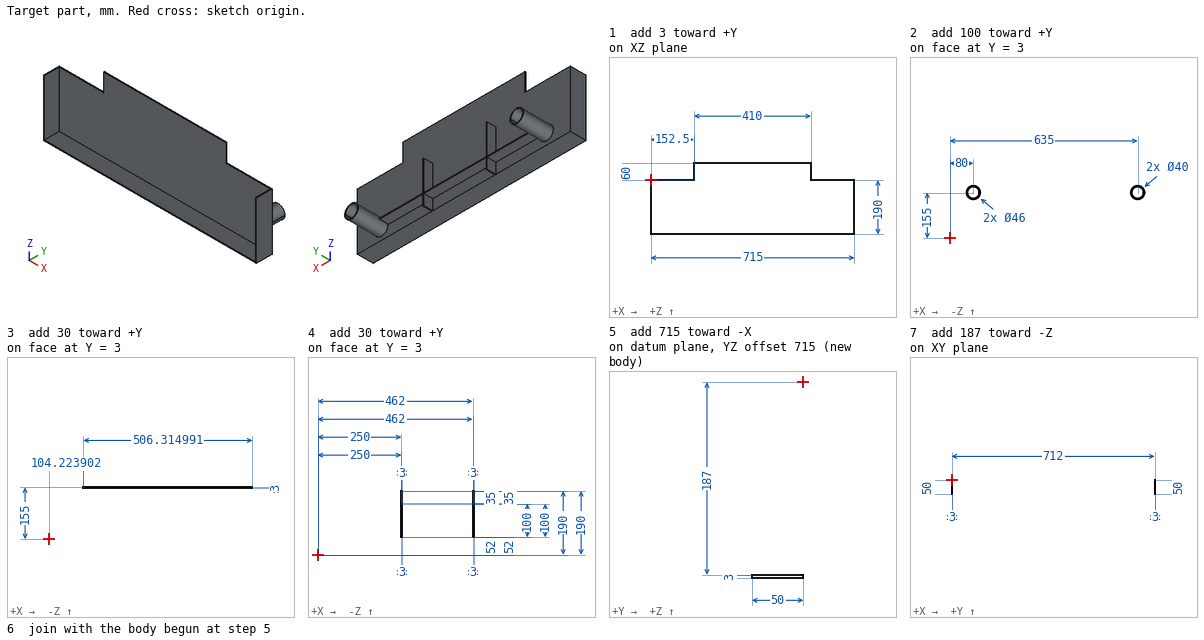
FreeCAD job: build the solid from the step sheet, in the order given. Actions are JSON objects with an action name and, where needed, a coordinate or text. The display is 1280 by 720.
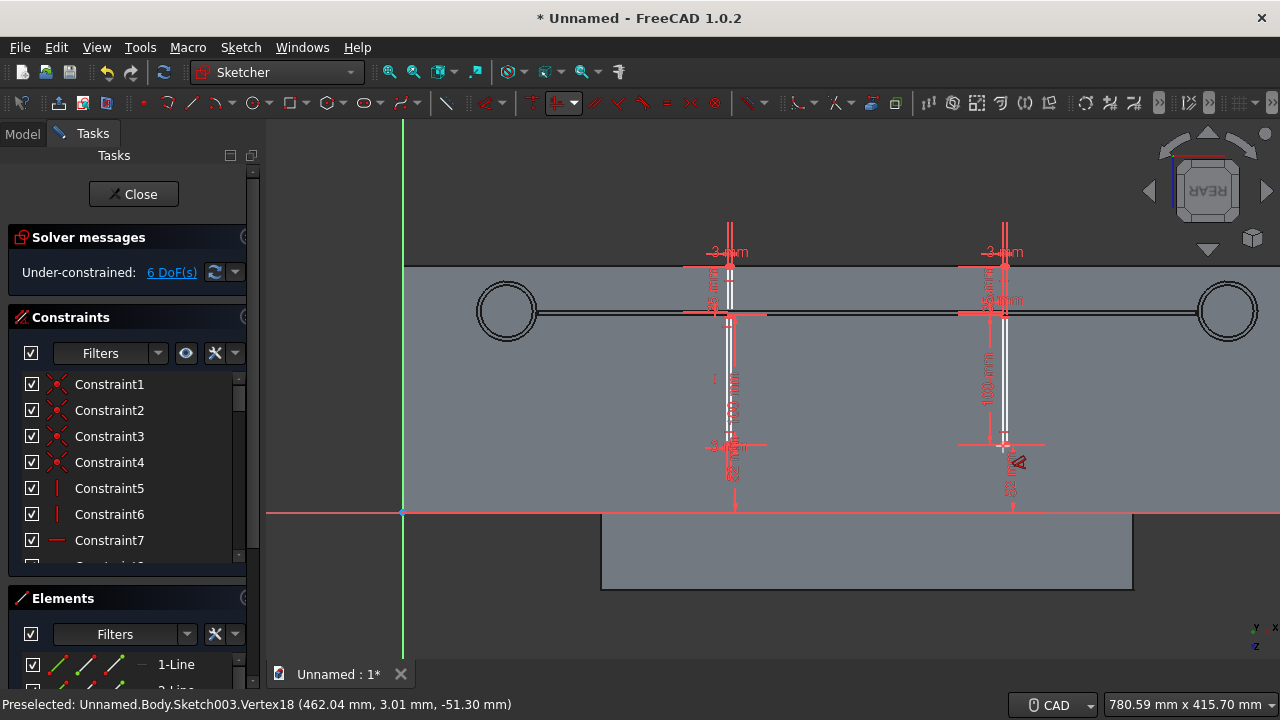
{"action": "scroll", "coordinate": [728, 267], "scroll_direction": "up", "scroll_amount": 6}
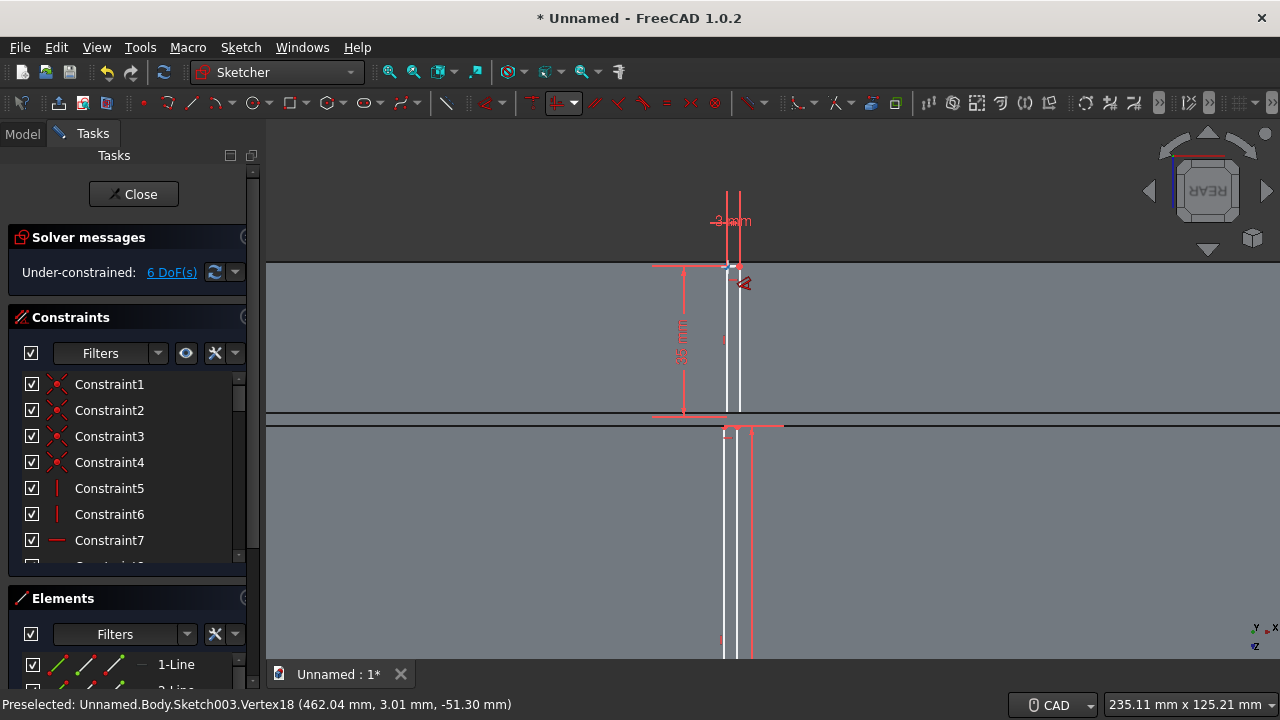
{"action": "left_click", "coordinate": [727, 266]}
{"action": "left_click", "coordinate": [510, 232]}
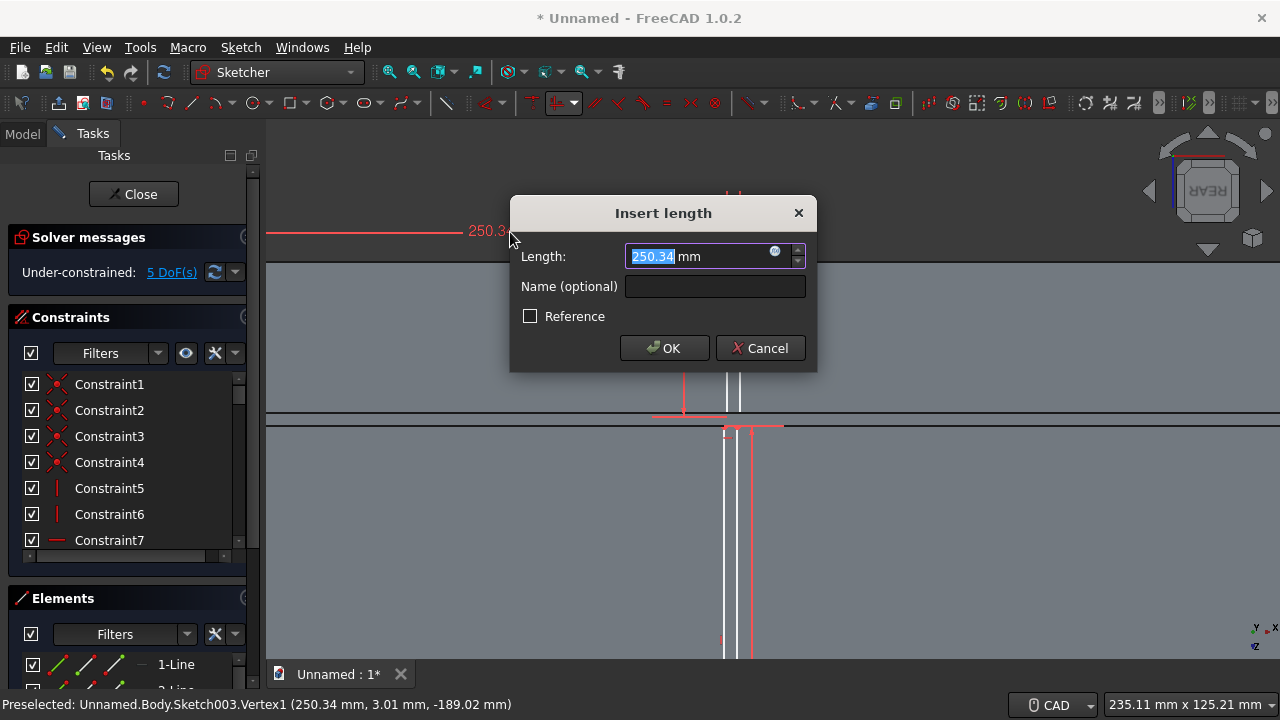
{"action": "type", "text": "250"}
{"action": "key", "text": "Return"}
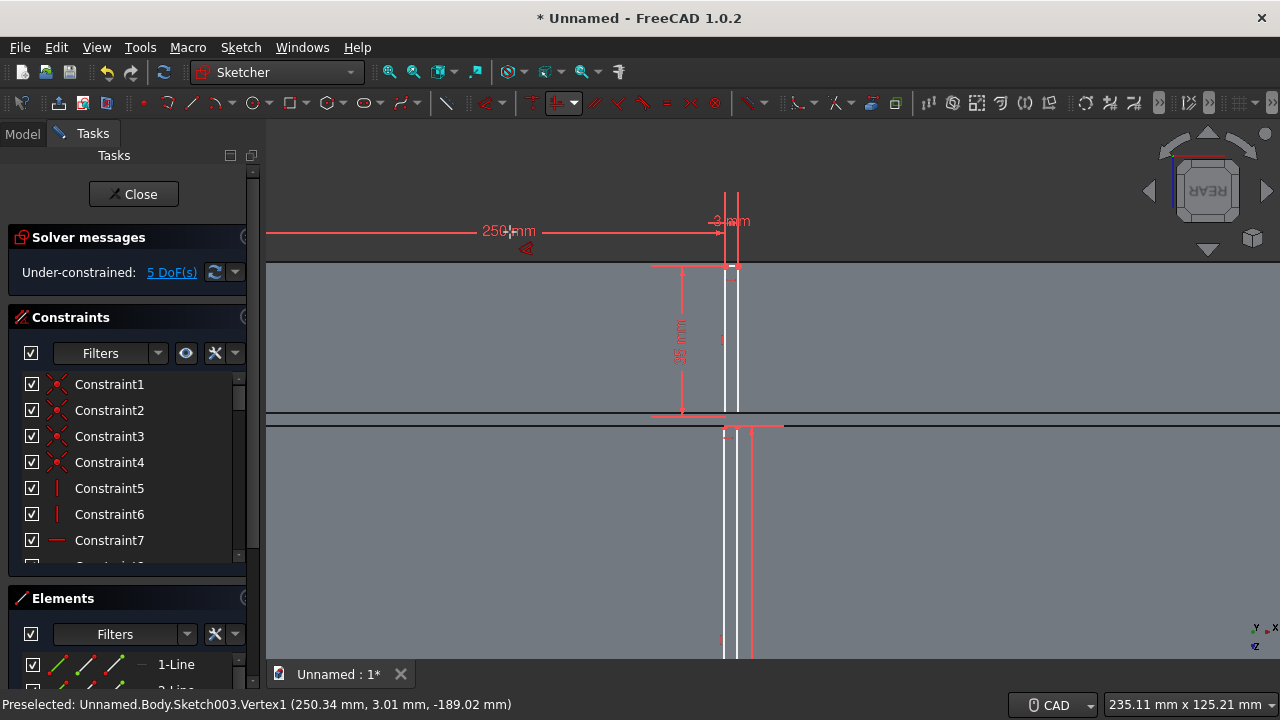
{"action": "left_click", "coordinate": [725, 266]}
{"action": "left_click", "coordinate": [759, 449]}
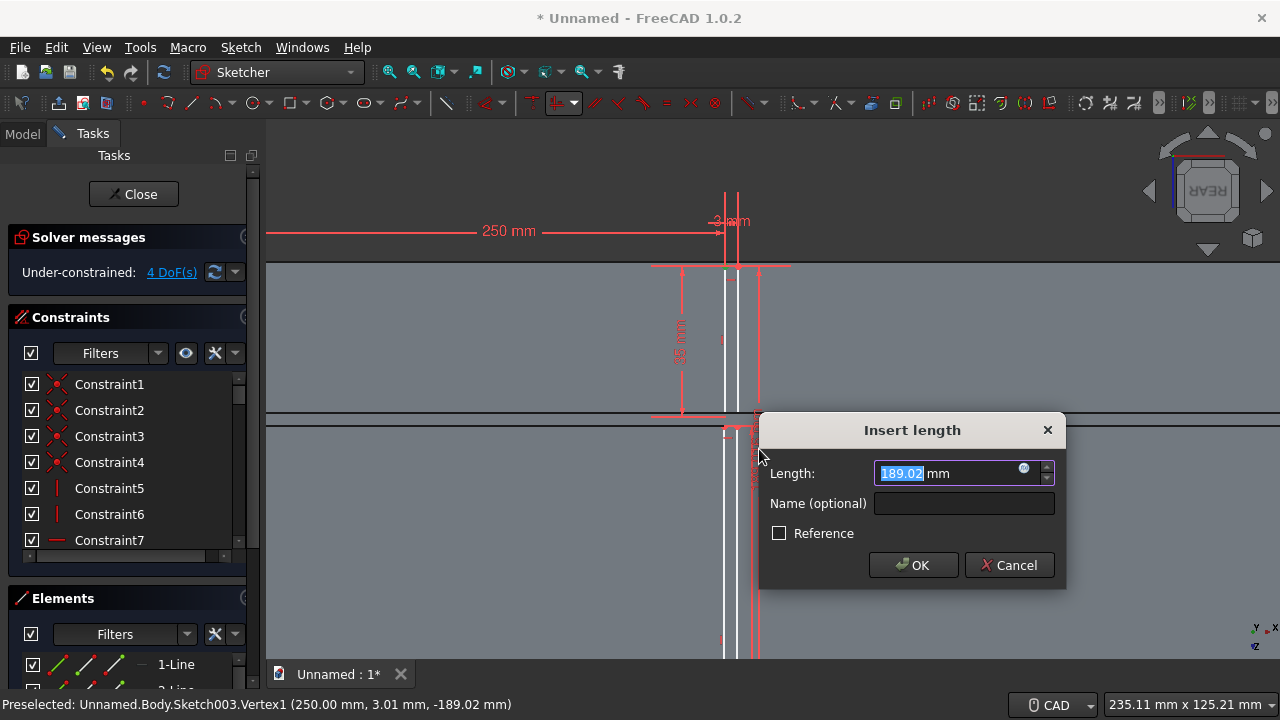
{"action": "type", "text": "190"}
{"action": "key", "text": "Return"}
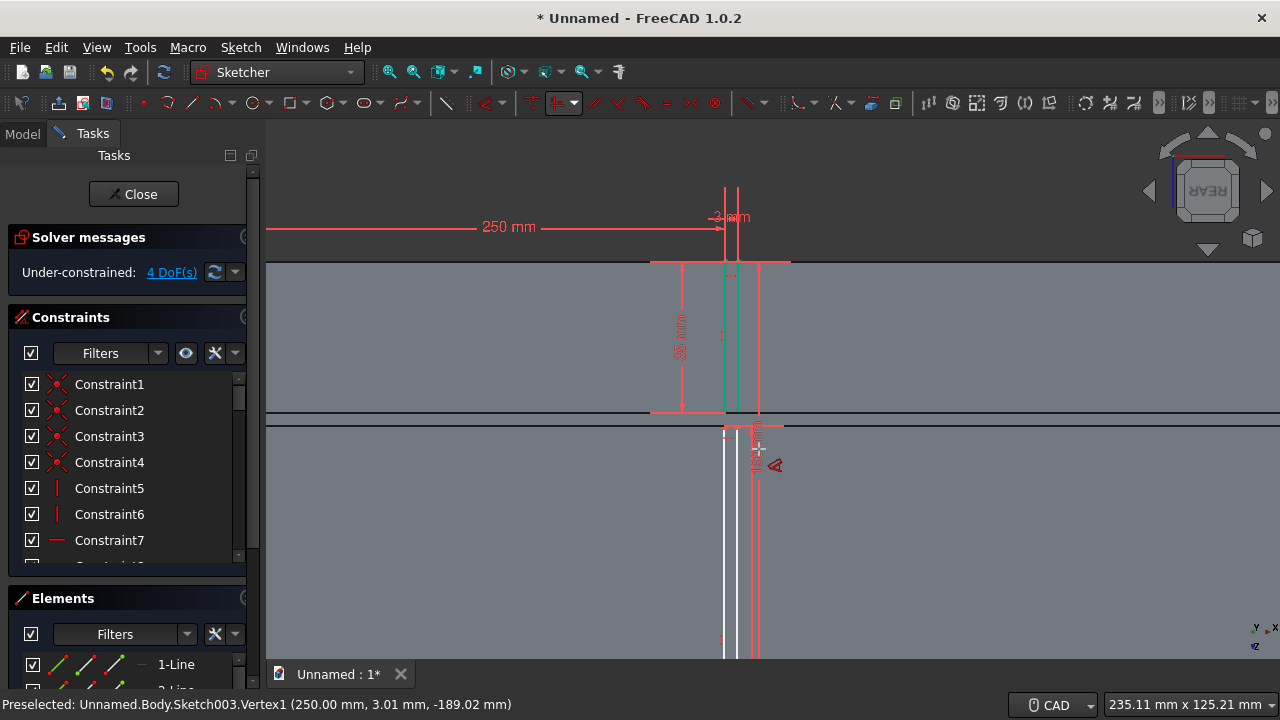
{"action": "left_click", "coordinate": [724, 426]}
{"action": "left_click", "coordinate": [509, 392]}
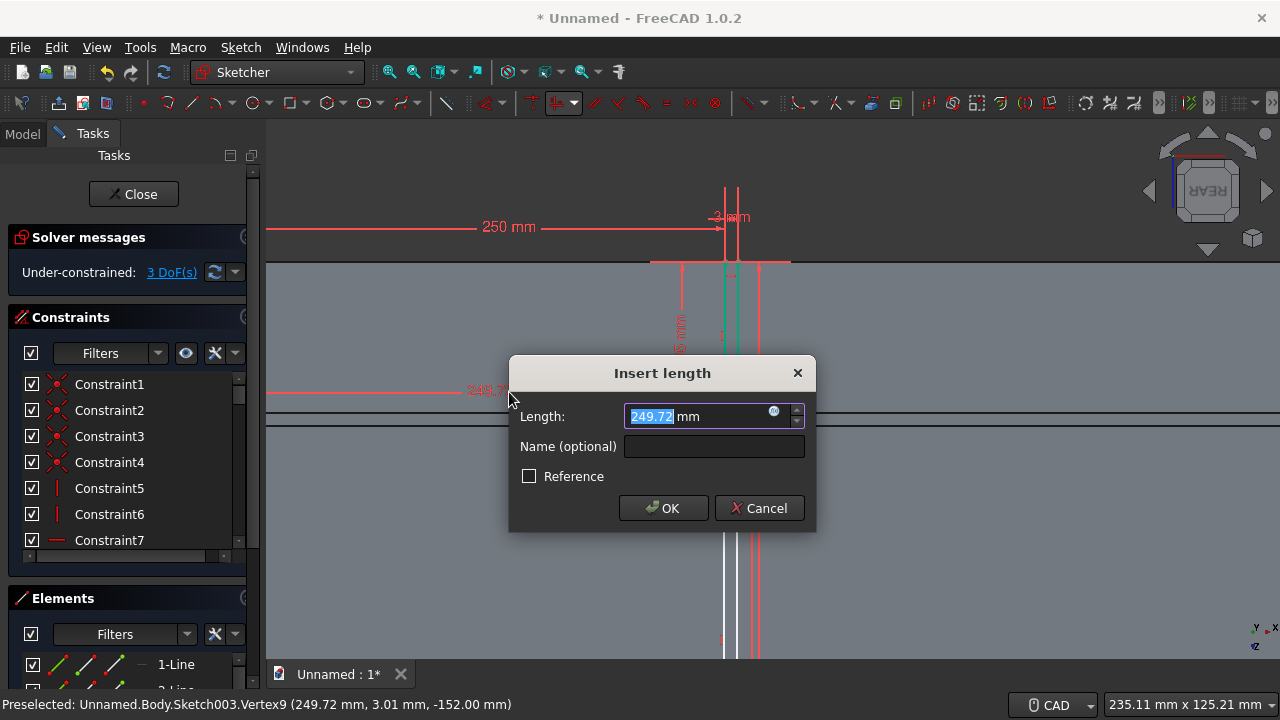
{"action": "type", "text": "250"}
{"action": "key", "text": "Return"}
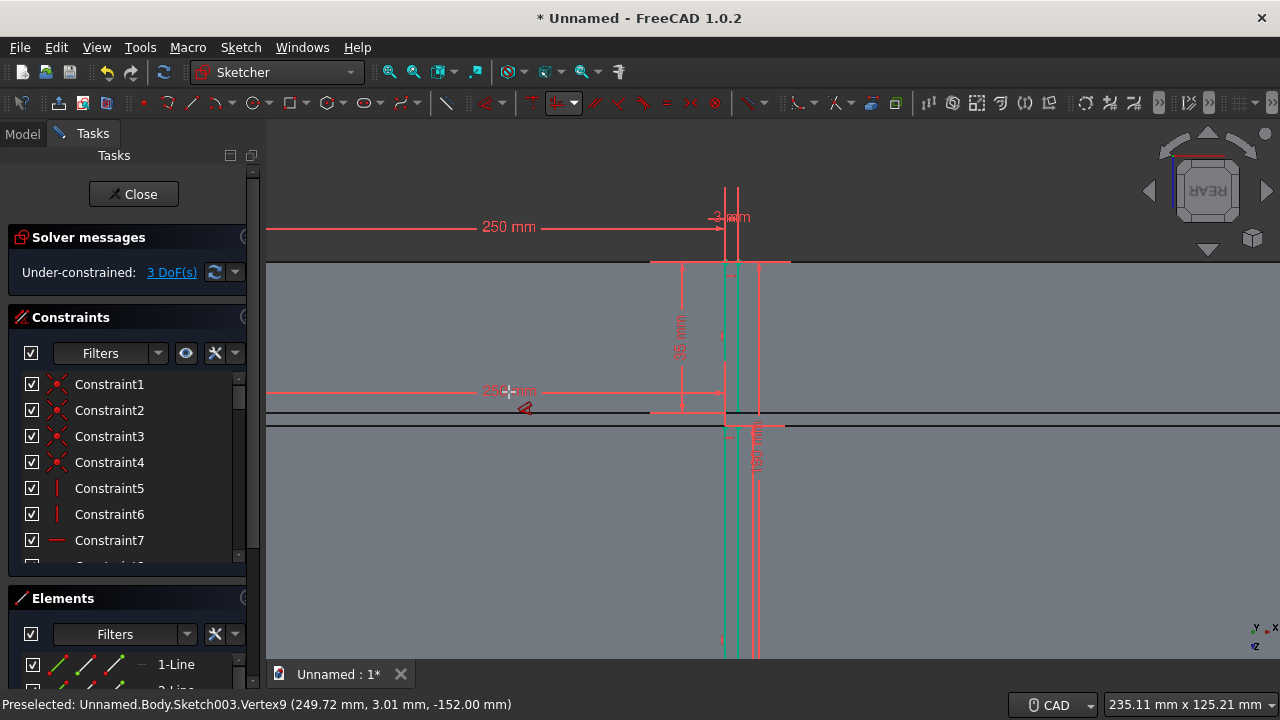
{"action": "scroll", "coordinate": [728, 267], "scroll_direction": "down", "scroll_amount": 6}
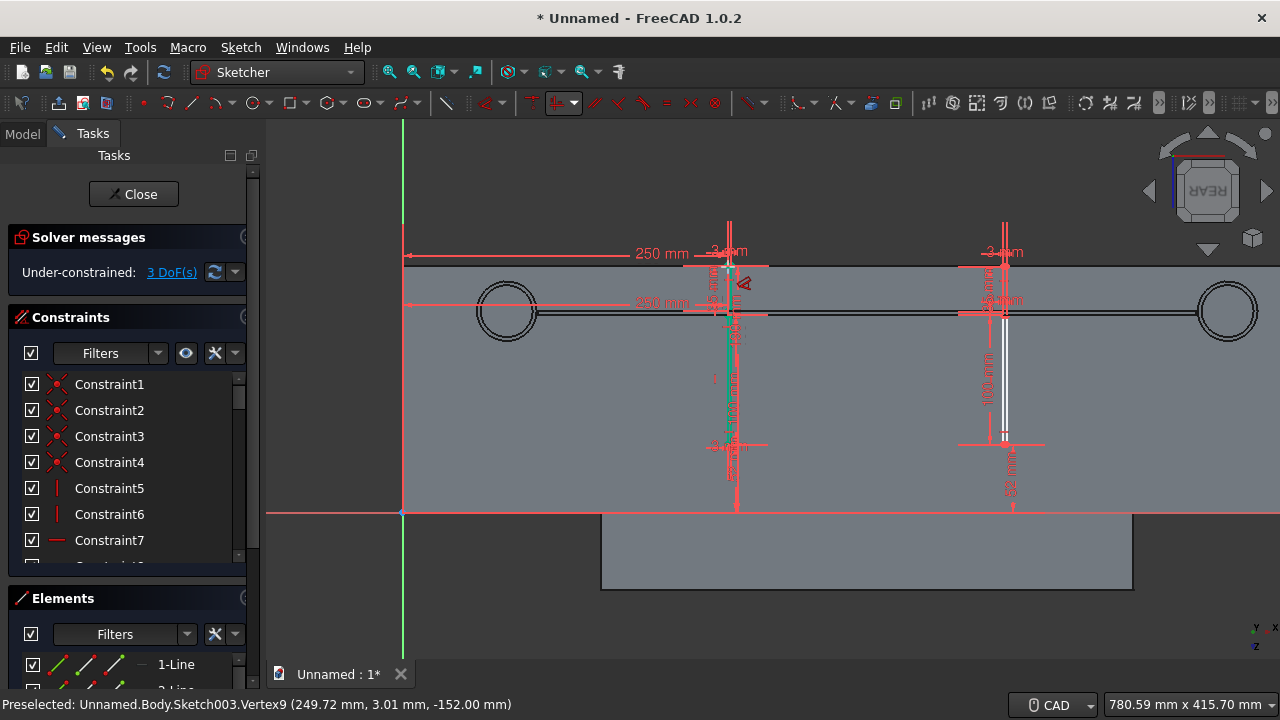
{"action": "scroll", "coordinate": [1003, 315], "scroll_direction": "up", "scroll_amount": 8}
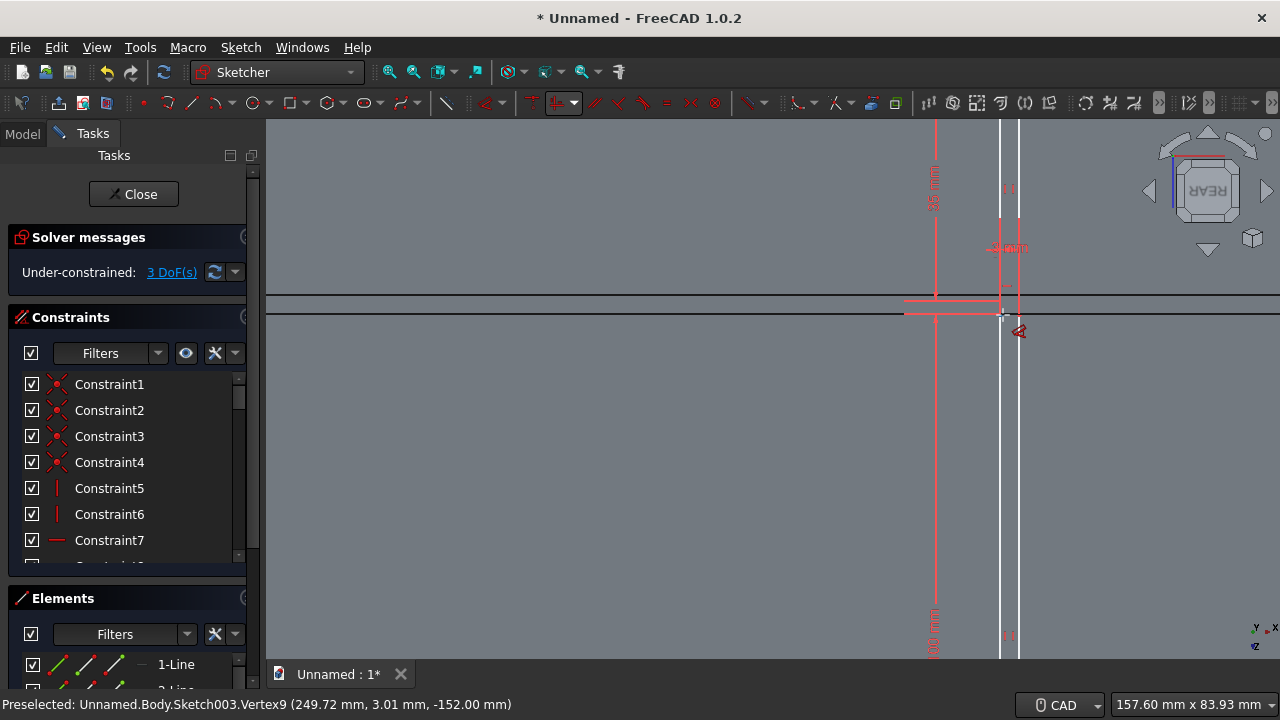
{"action": "left_click", "coordinate": [1000, 314]}
{"action": "left_click", "coordinate": [647, 280]}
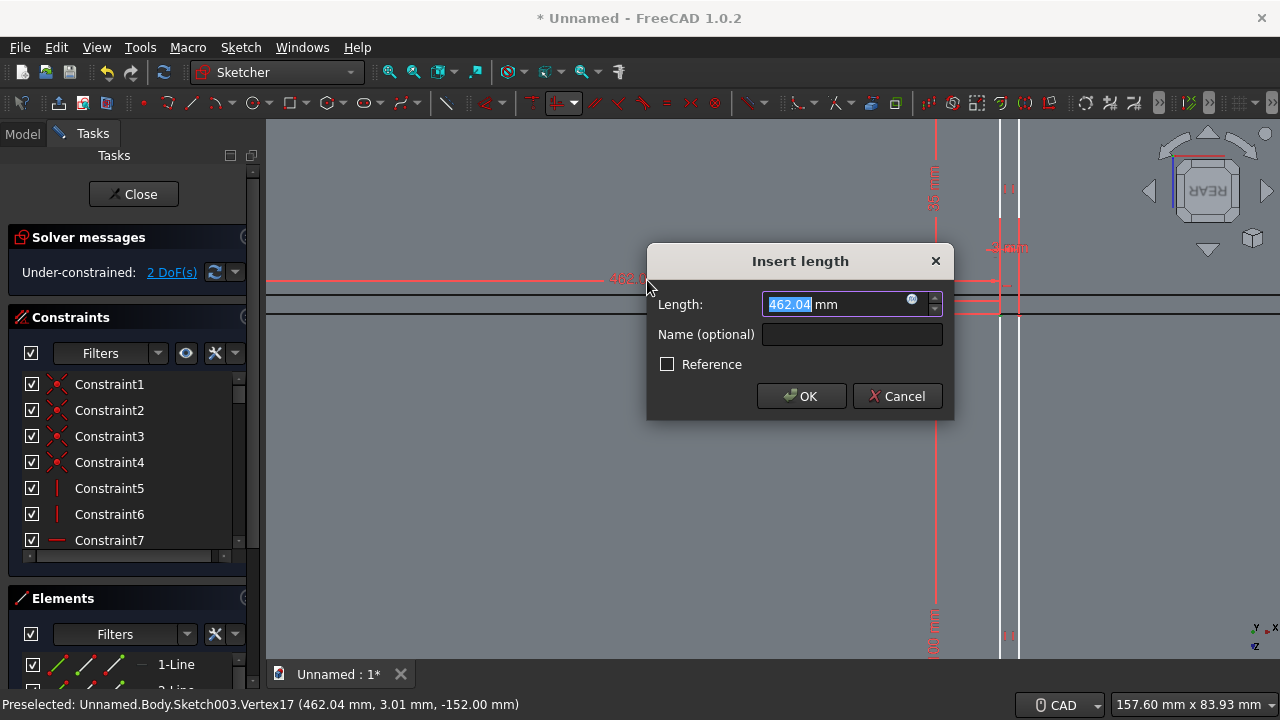
{"action": "type", "text": "462"}
{"action": "key", "text": "Return"}